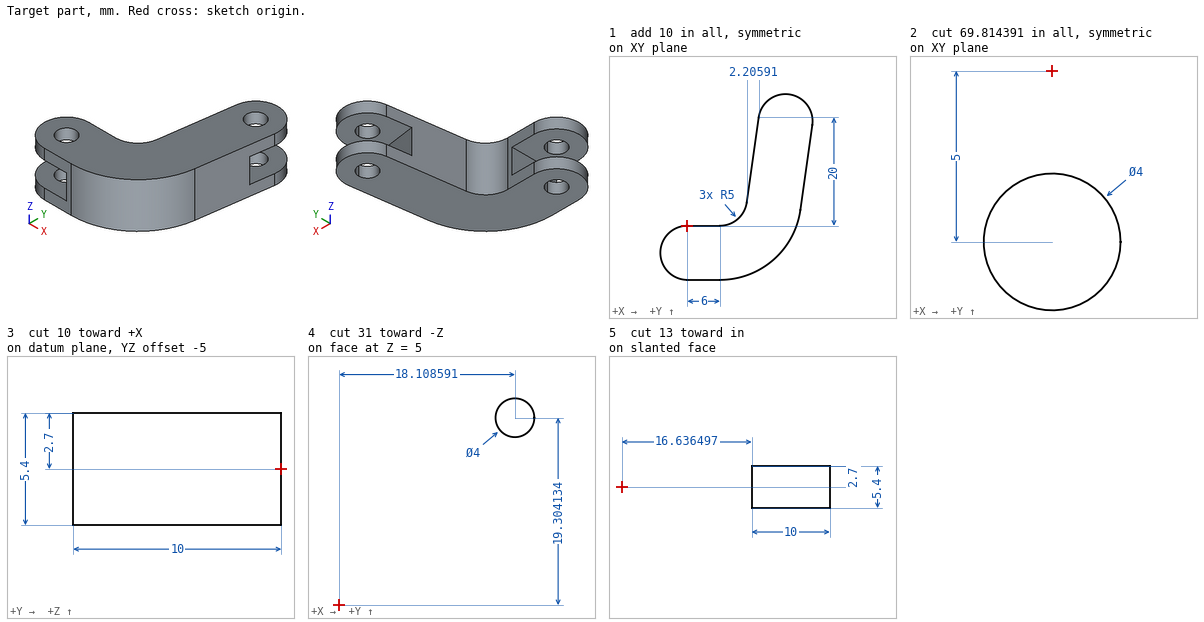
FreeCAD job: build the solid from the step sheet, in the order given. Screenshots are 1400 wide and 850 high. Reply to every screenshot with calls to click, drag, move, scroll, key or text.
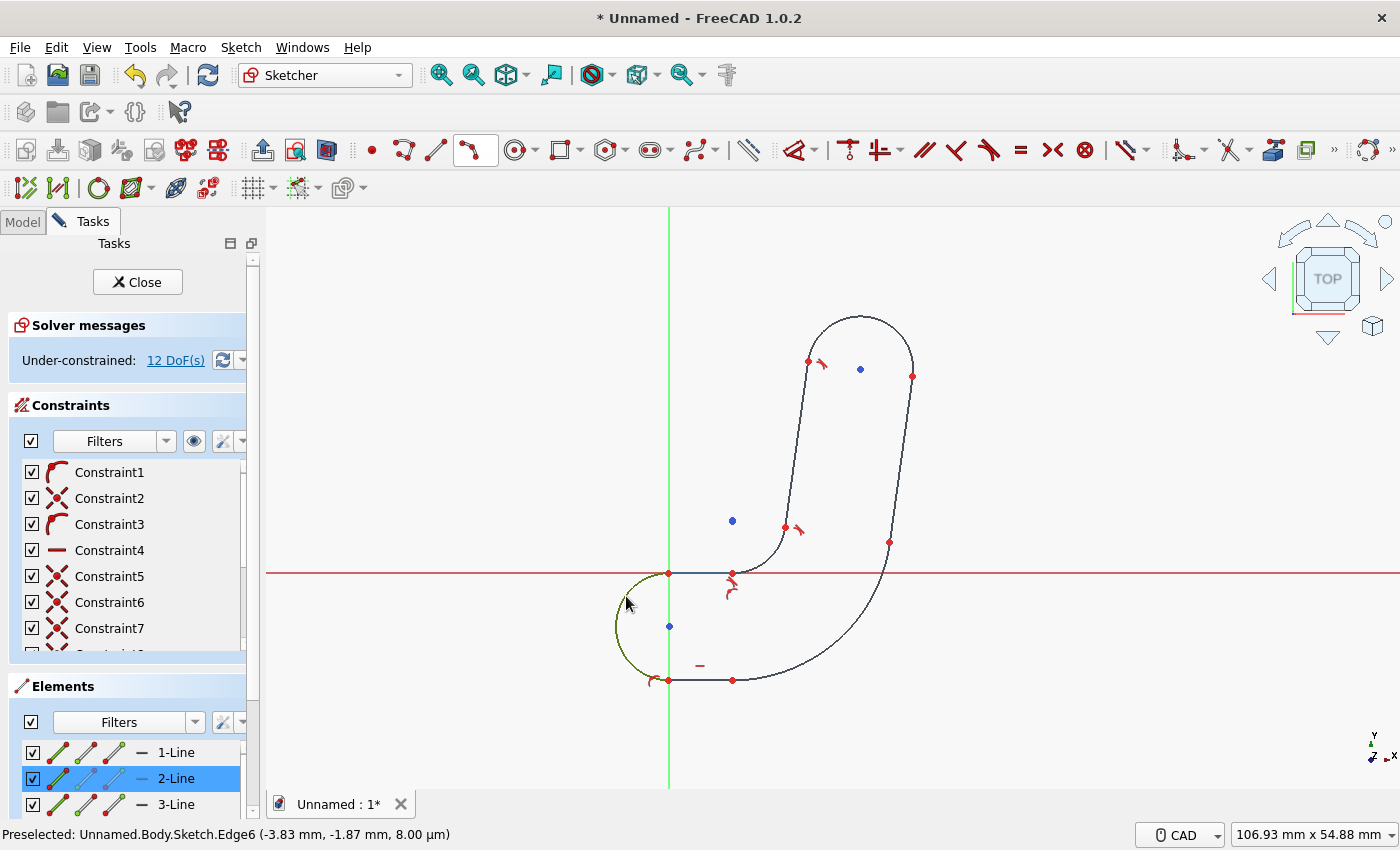
click(990, 150)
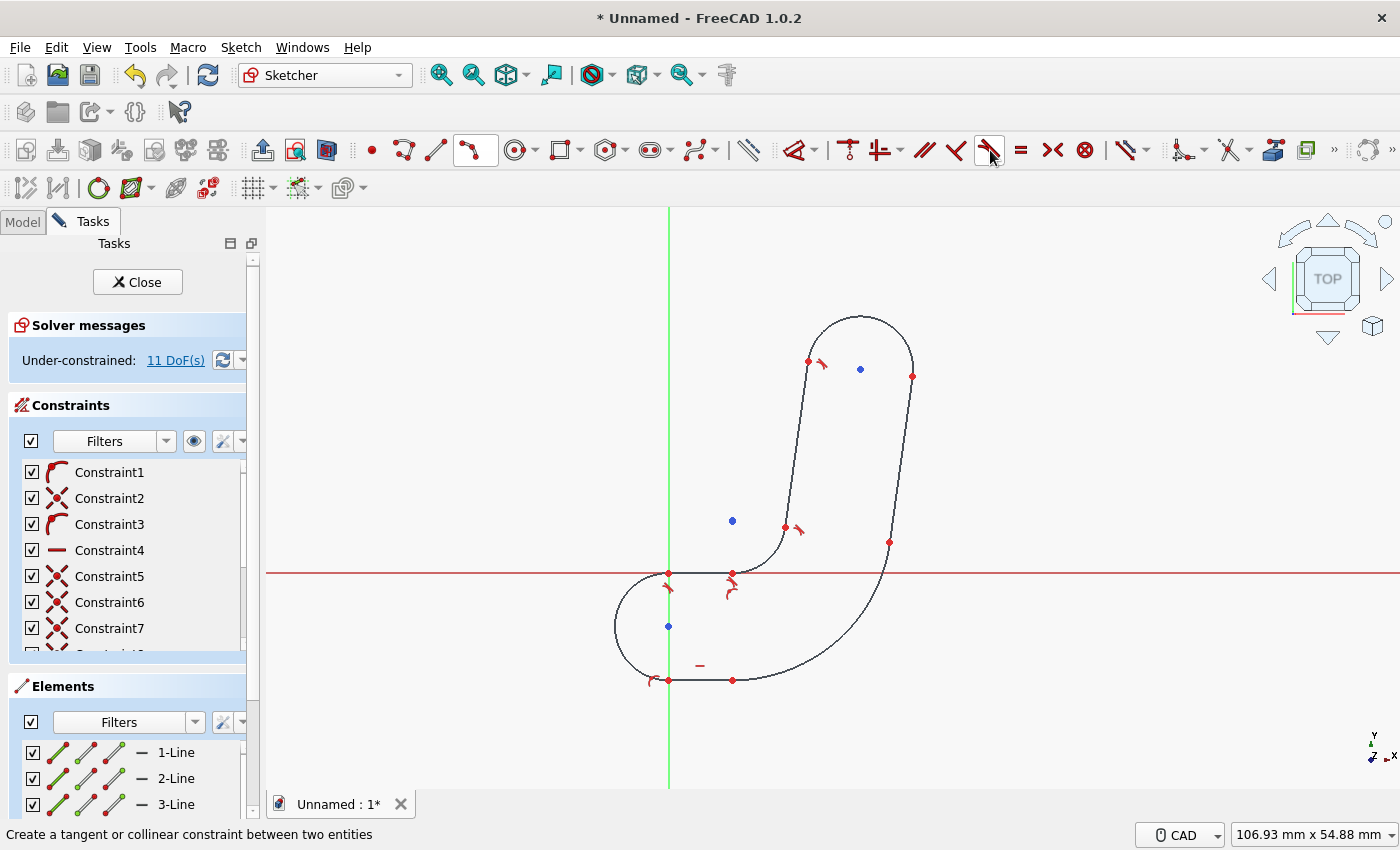
click(688, 680)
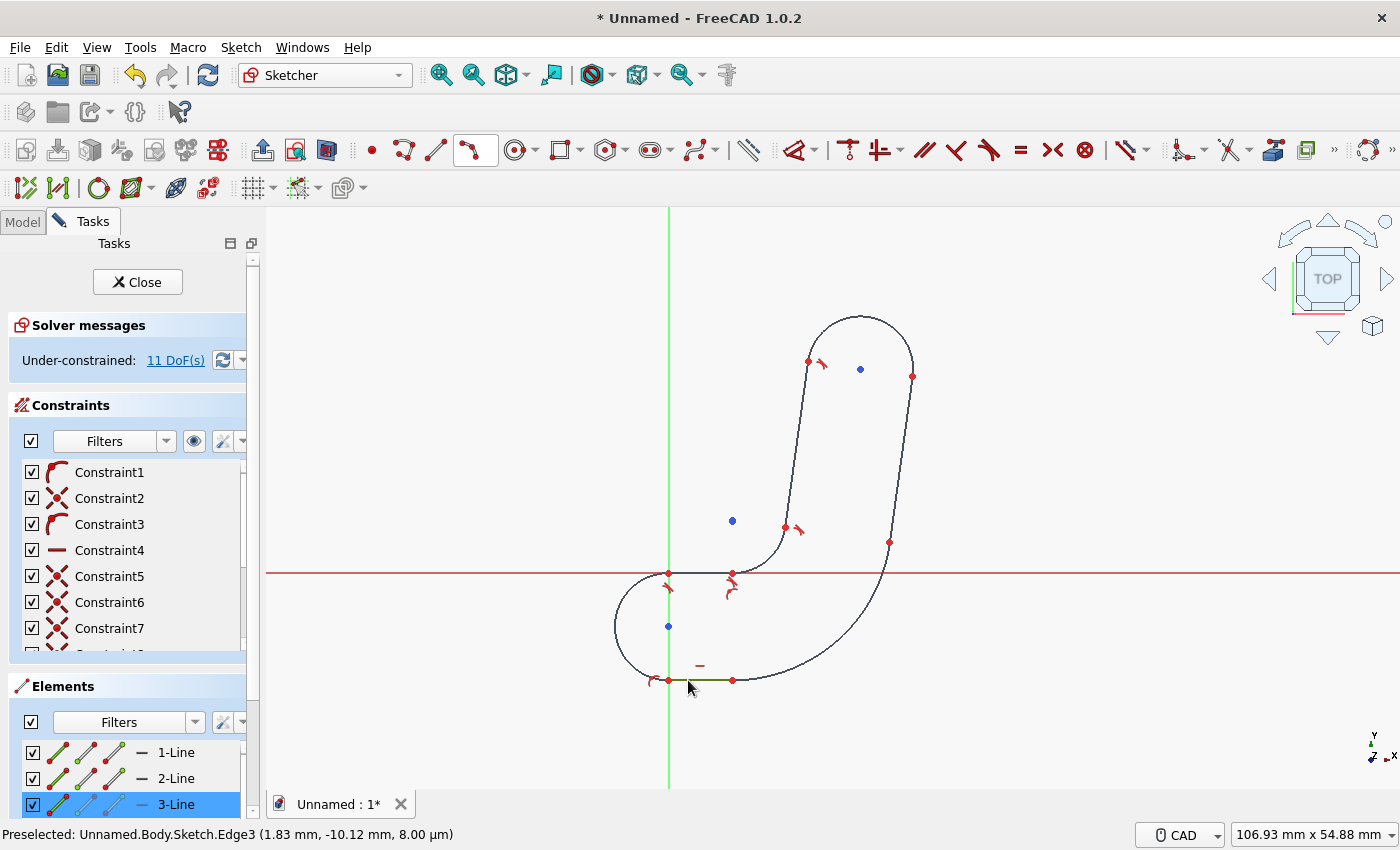
click(799, 666)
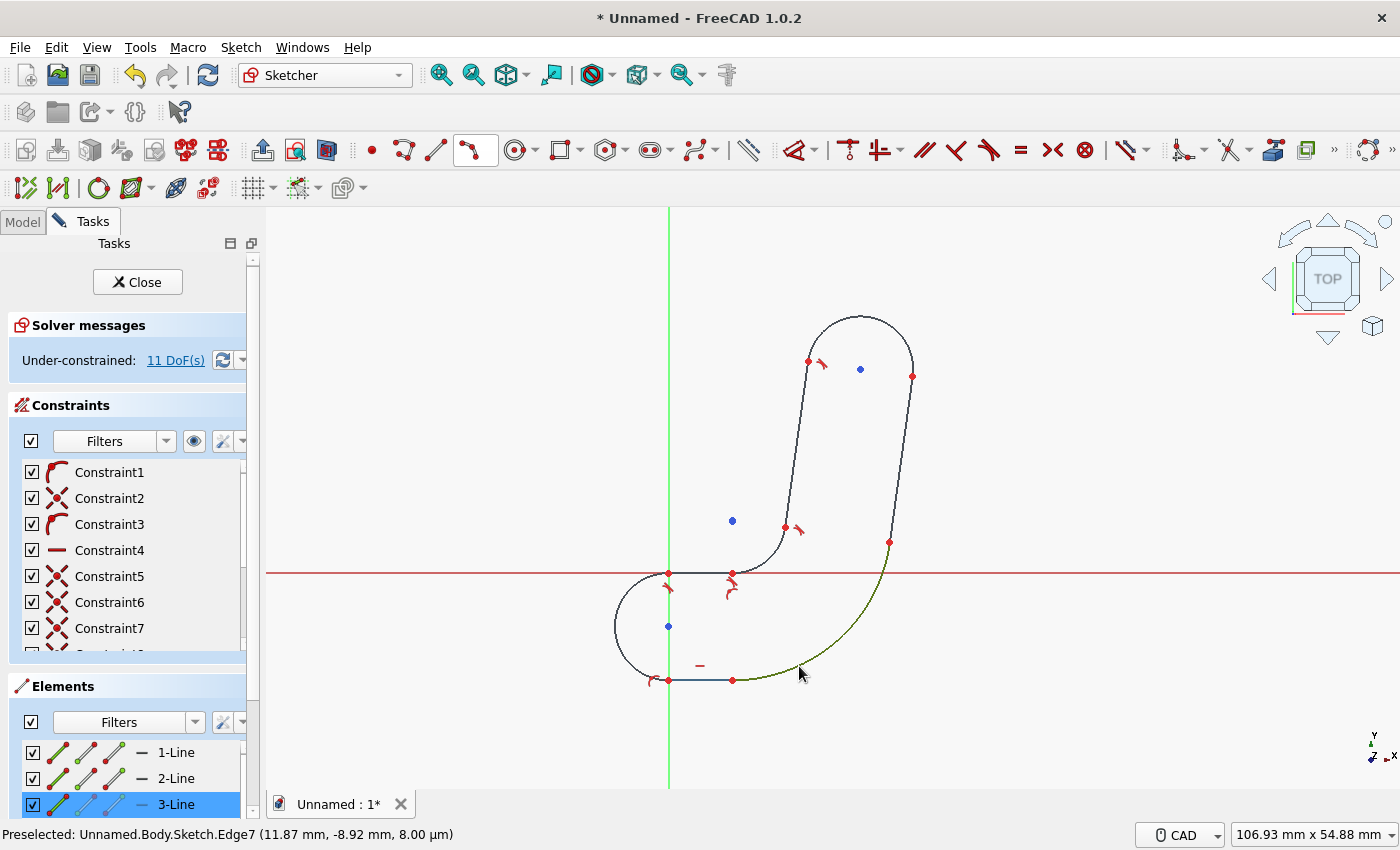
click(990, 150)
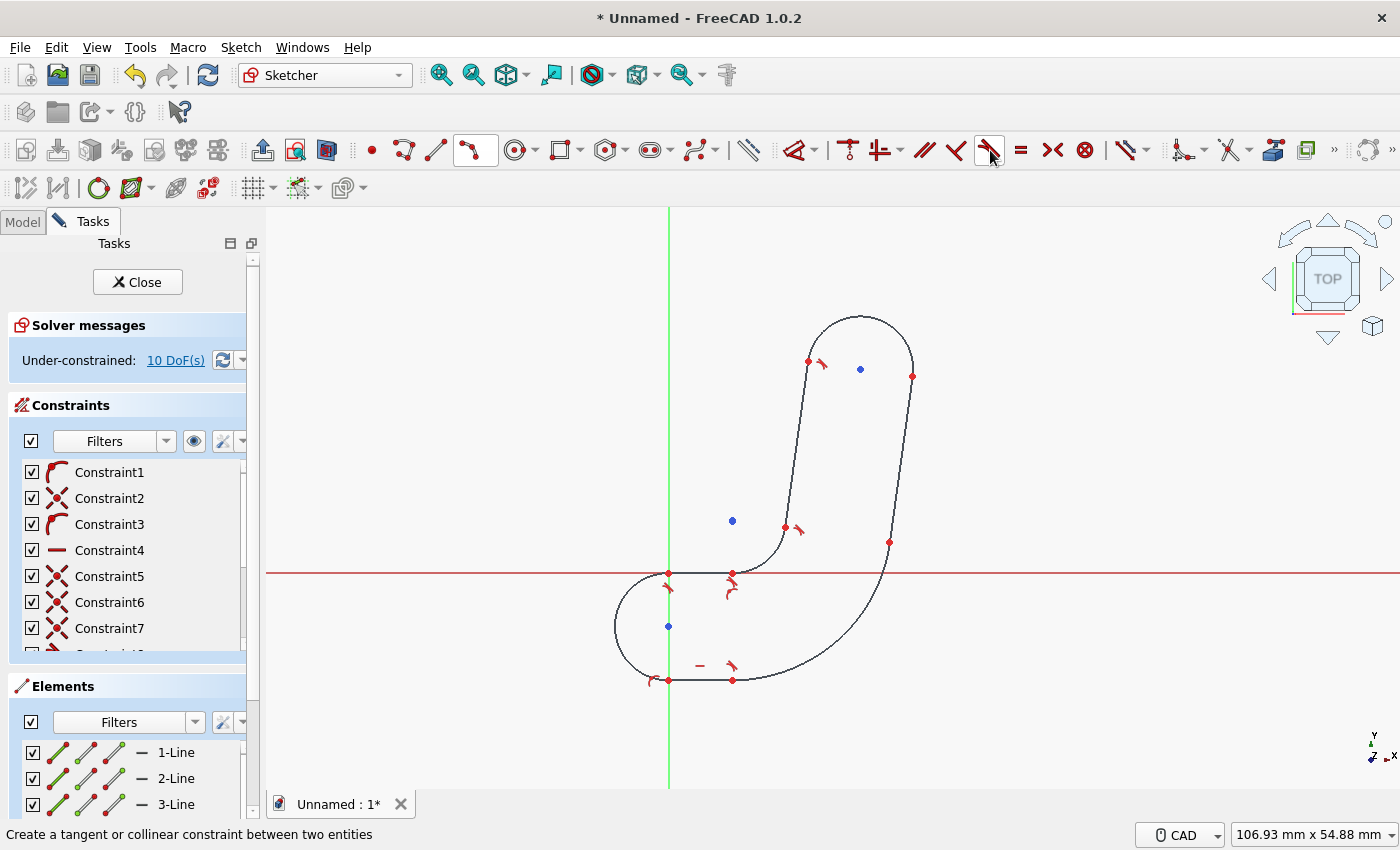
click(897, 493)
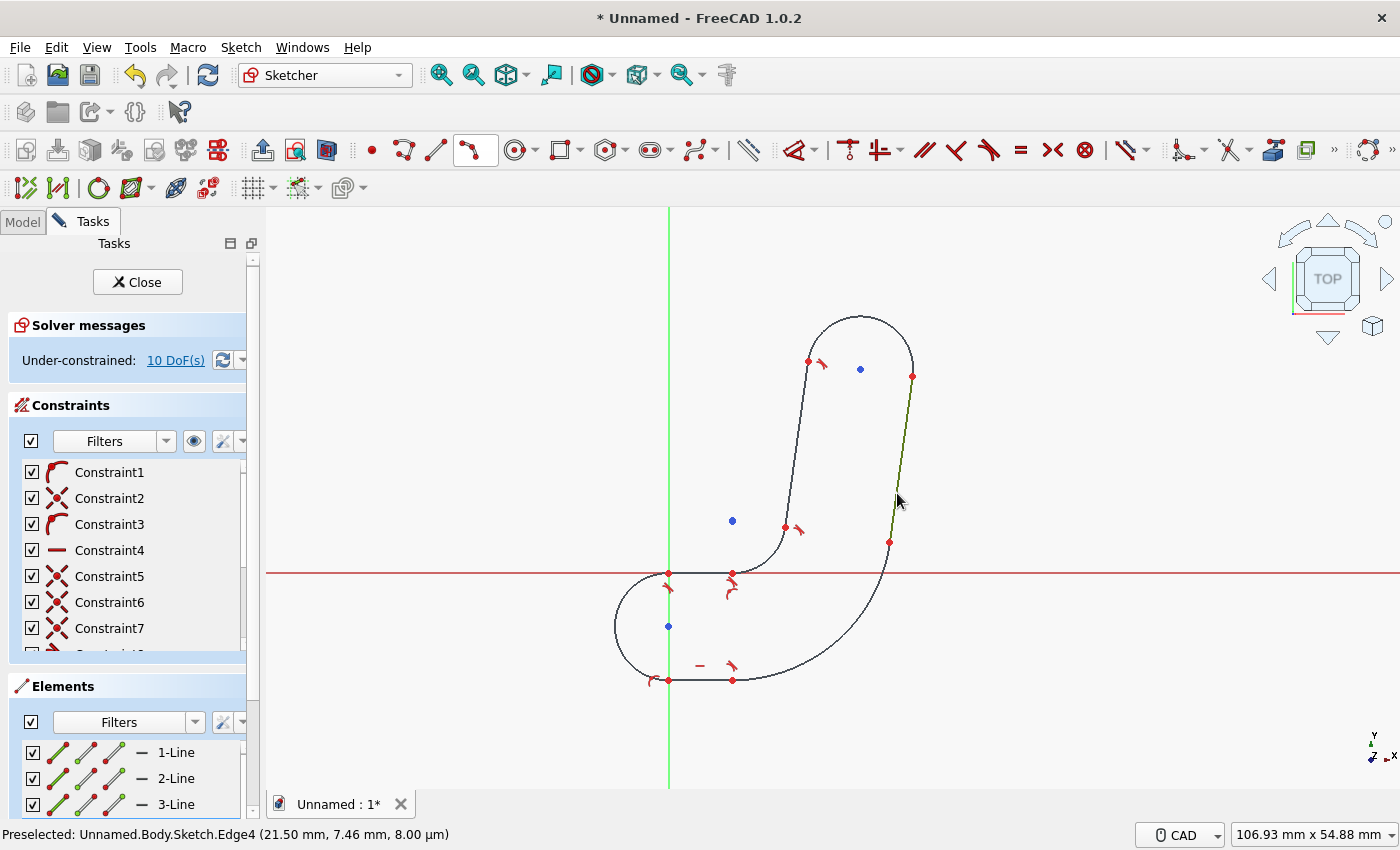
click(799, 666)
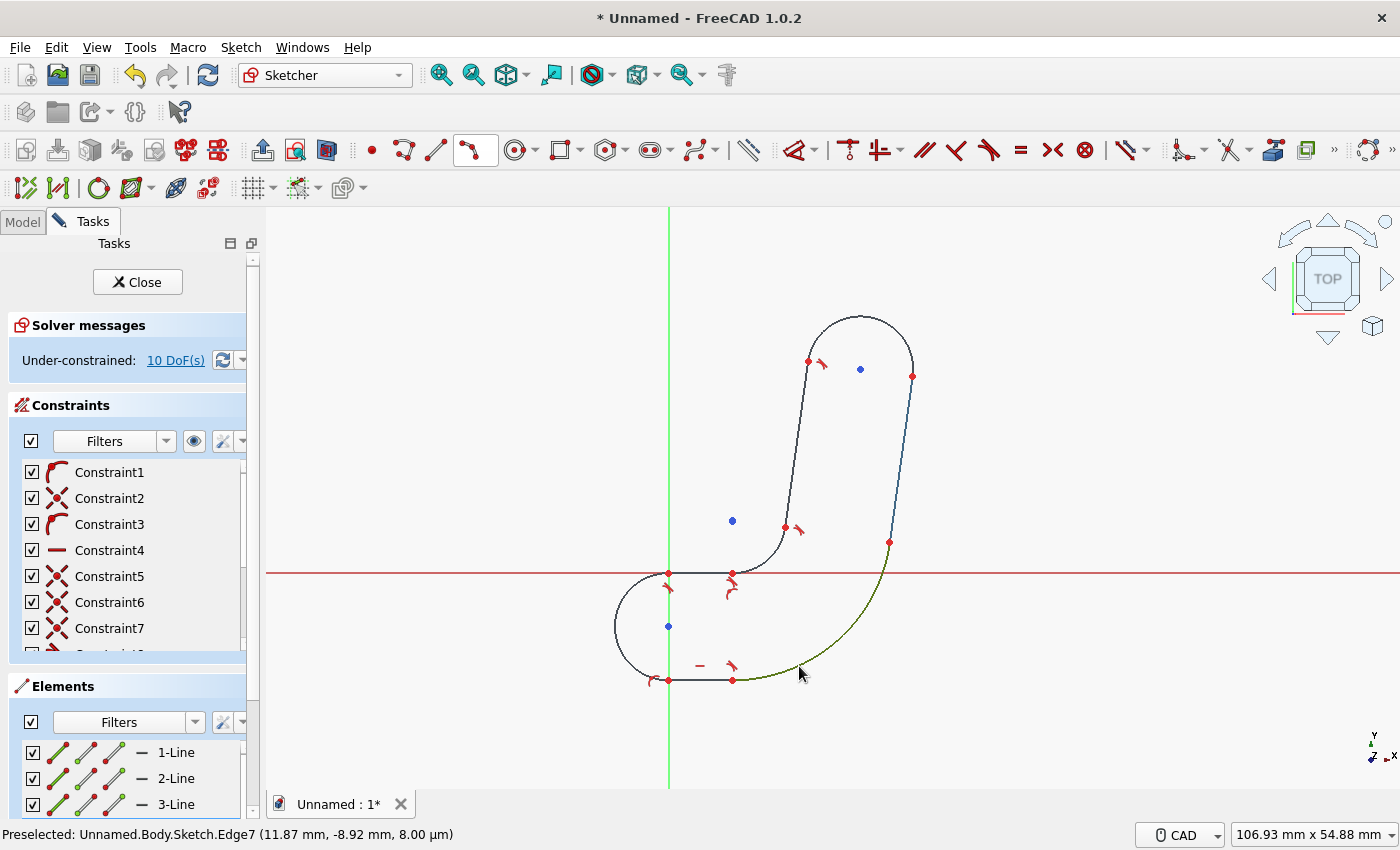
click(990, 150)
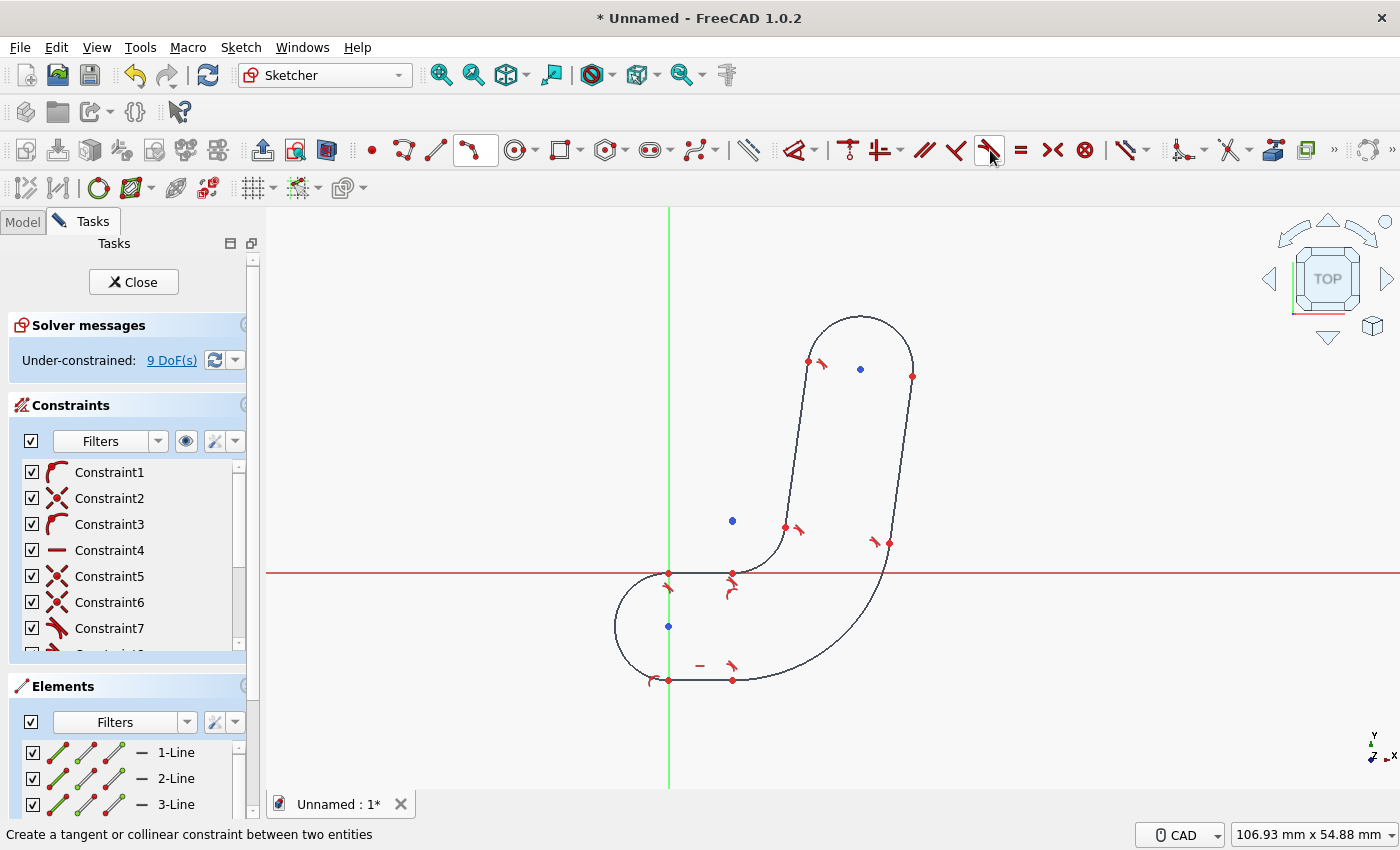
click(897, 493)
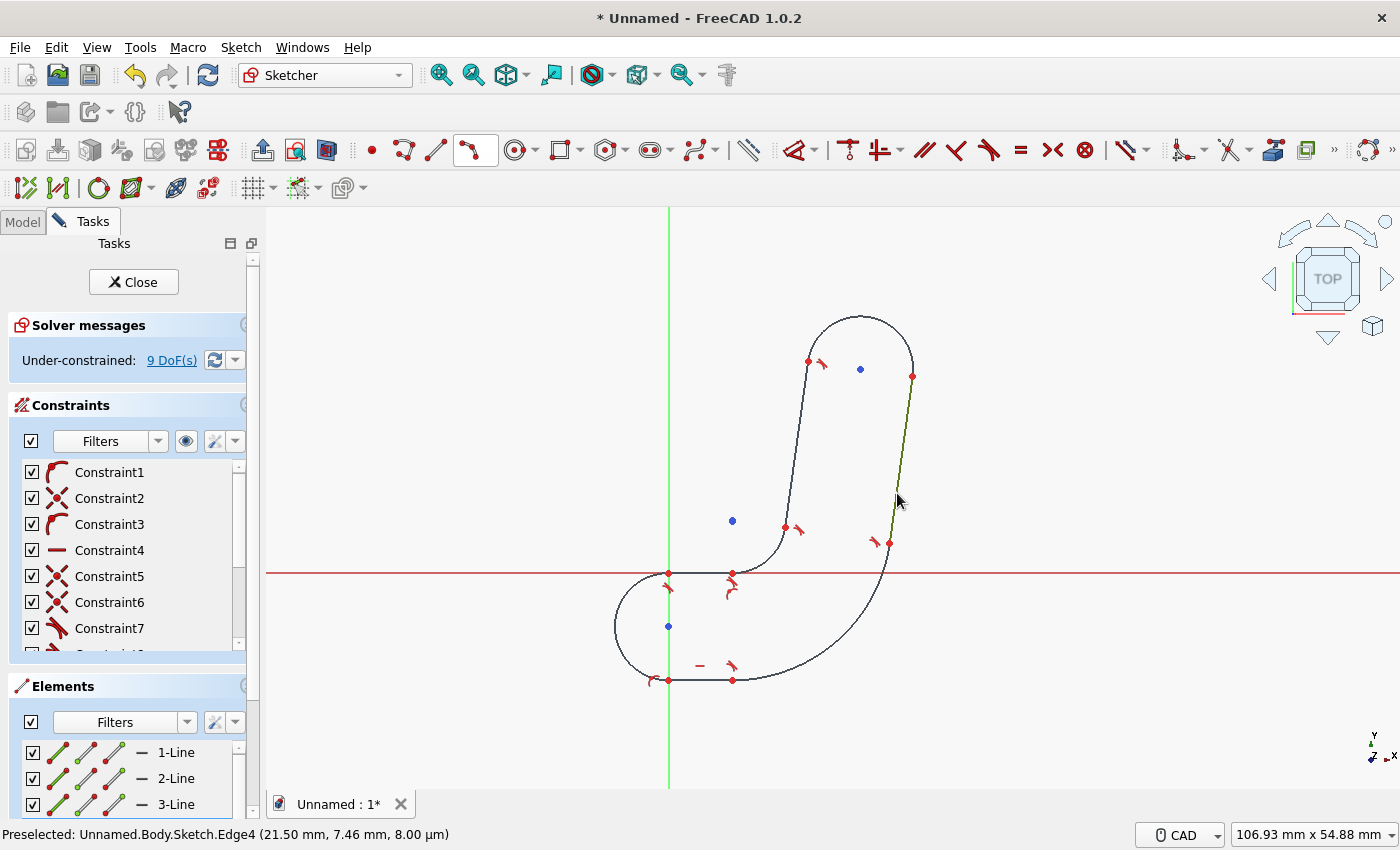
click(897, 331)